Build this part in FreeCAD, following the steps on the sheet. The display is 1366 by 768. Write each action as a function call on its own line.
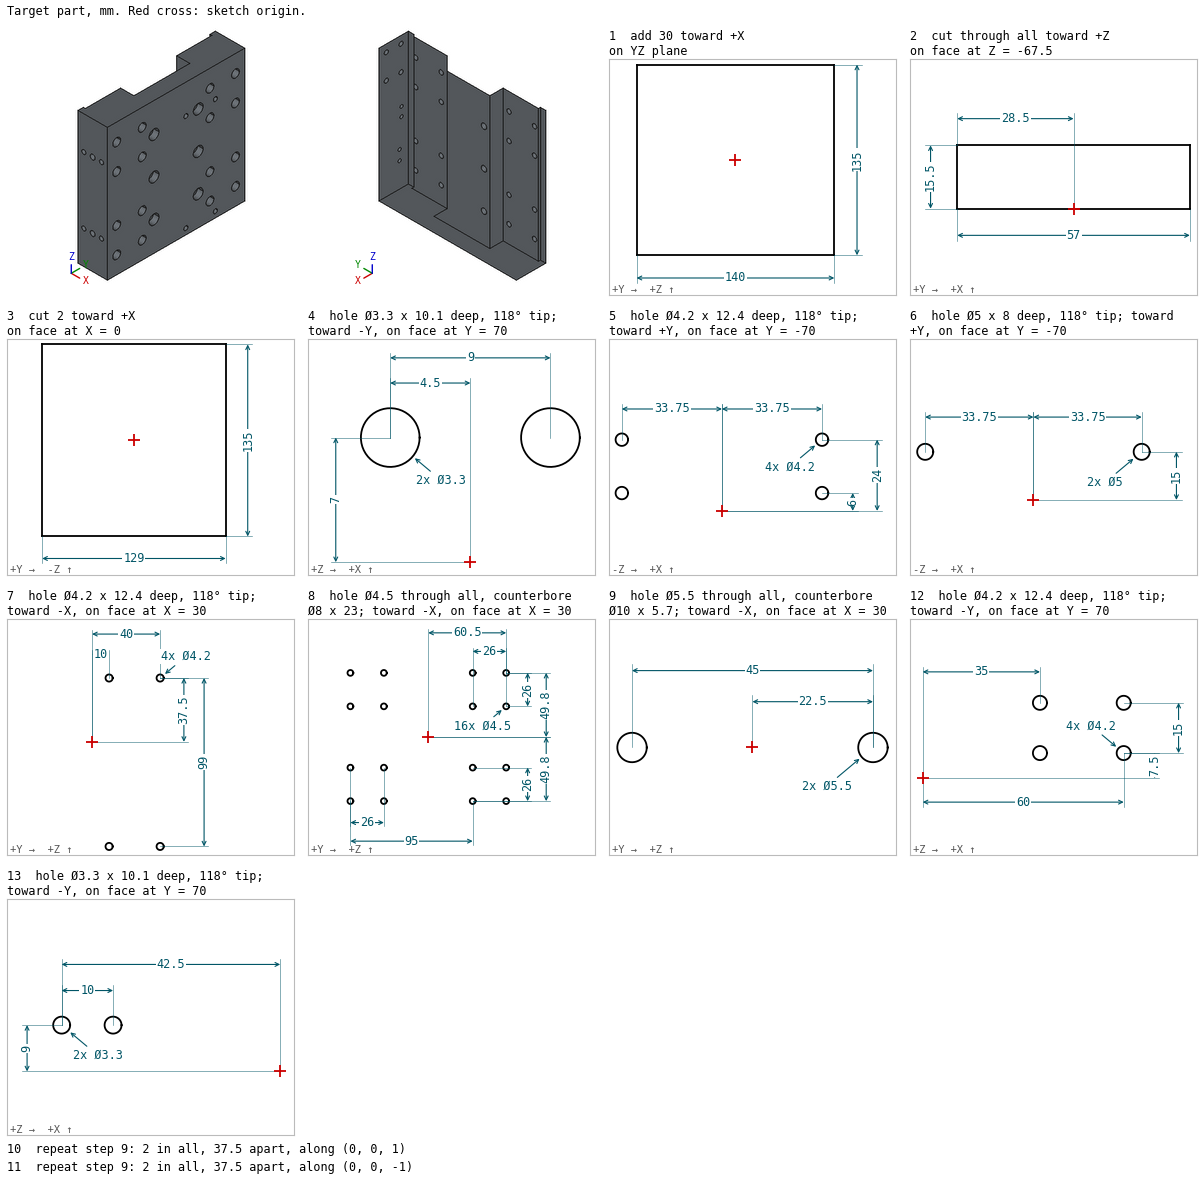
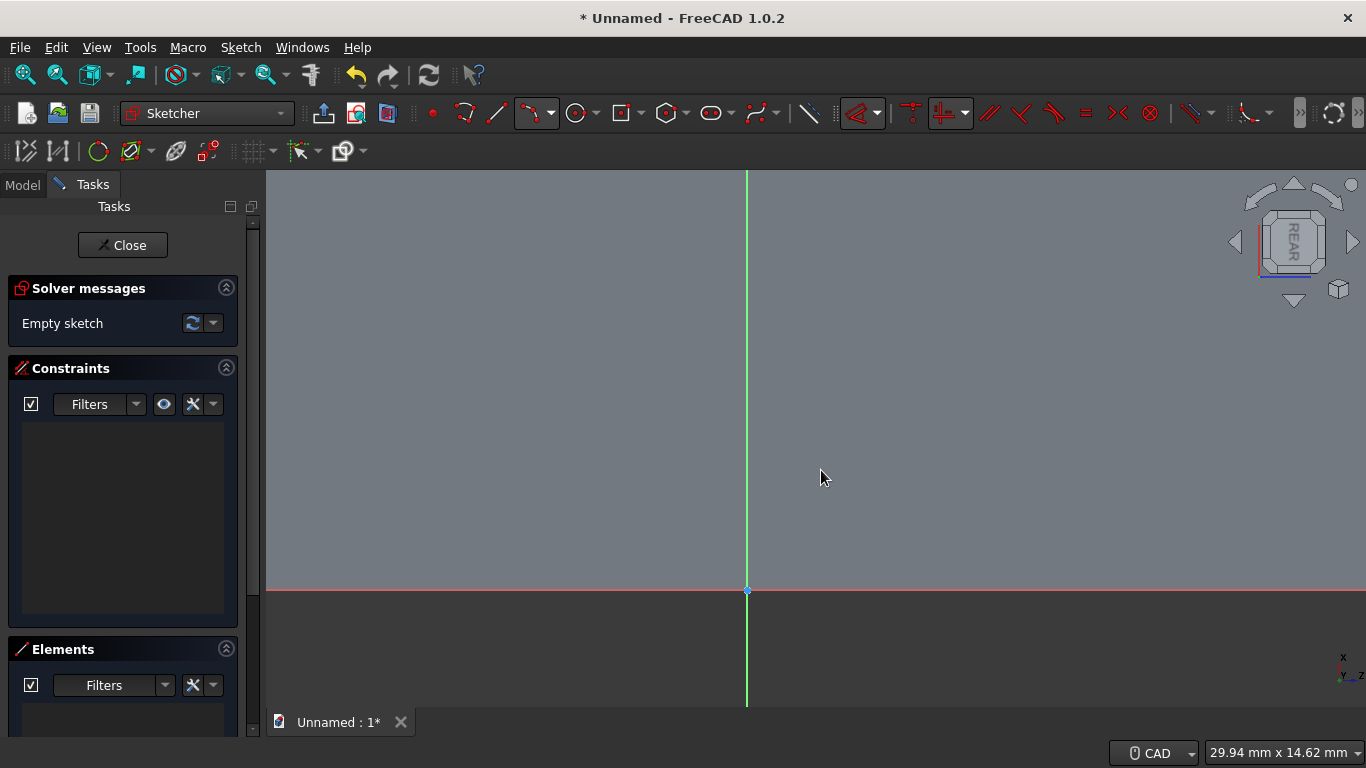
click(576, 114)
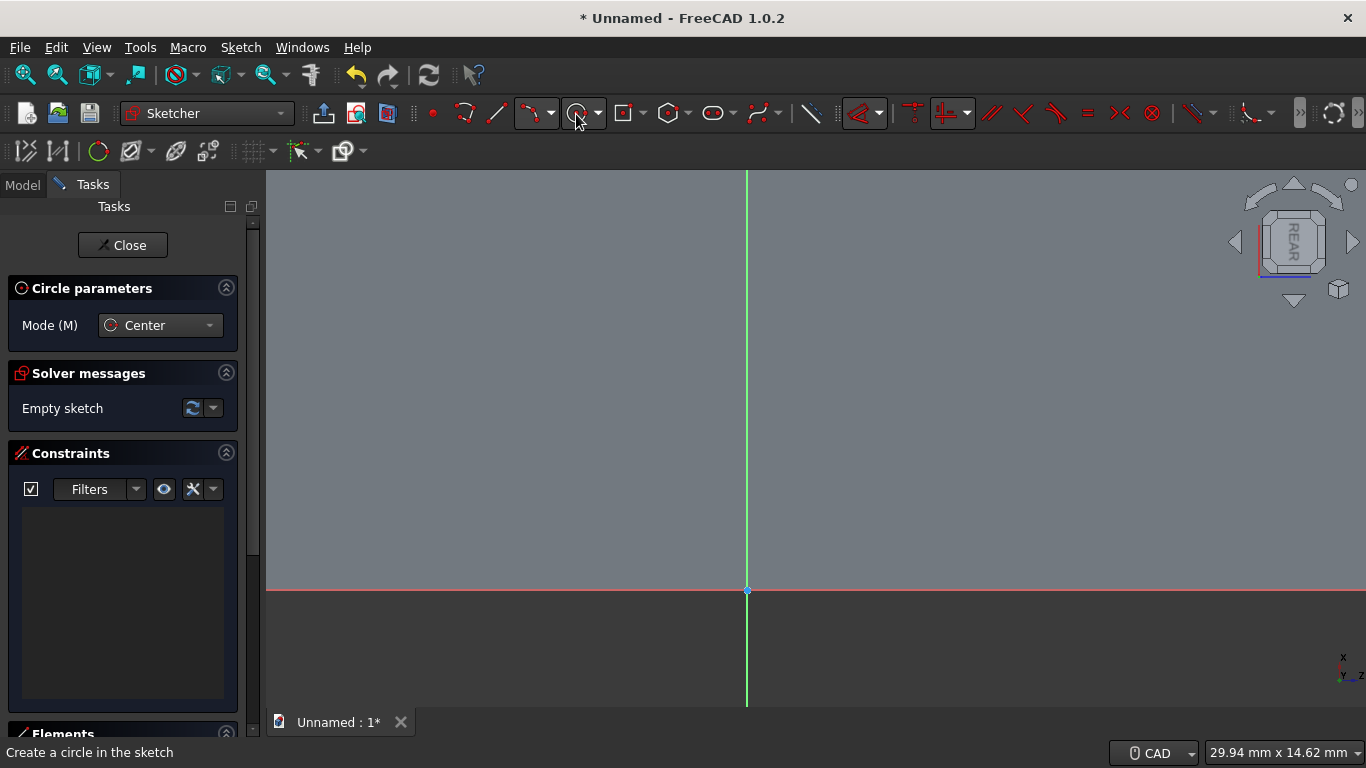
click(582, 333)
click(625, 290)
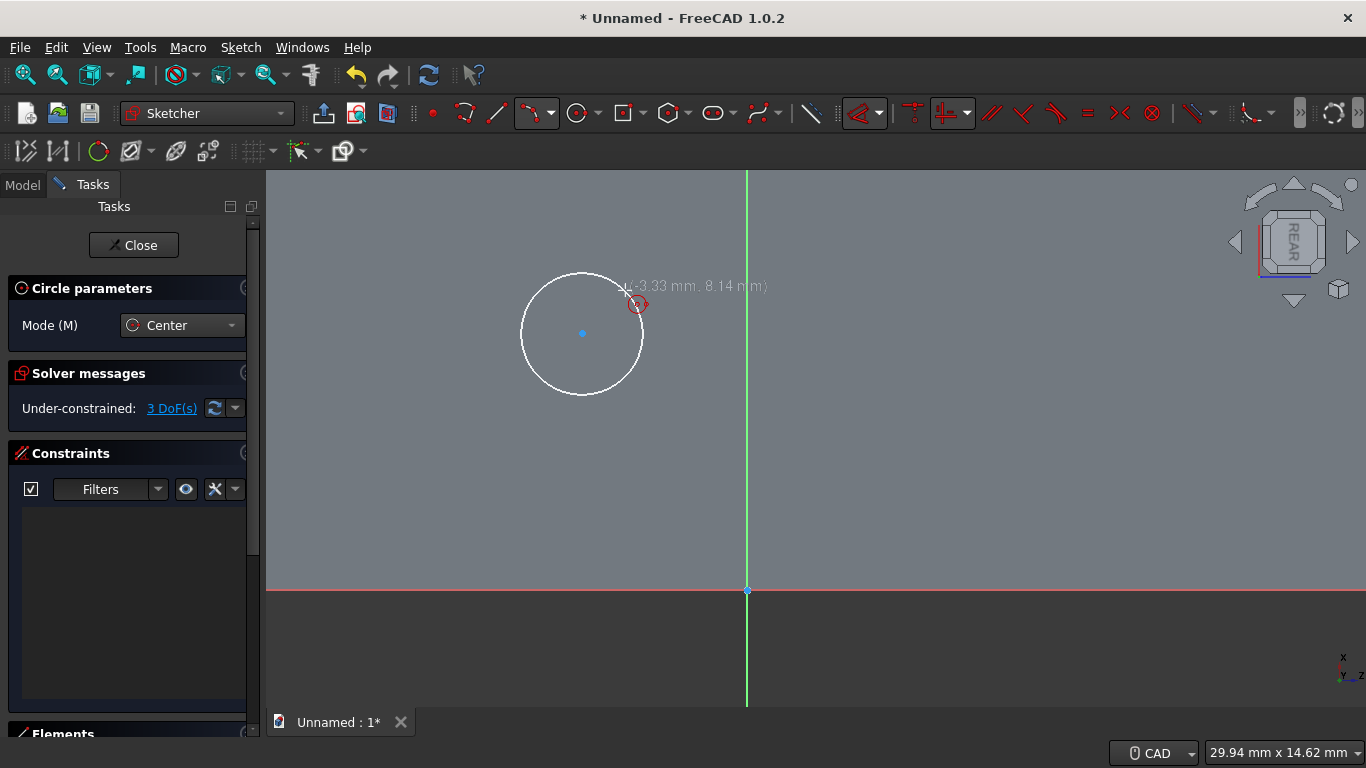
click(913, 333)
click(956, 290)
key(Escape)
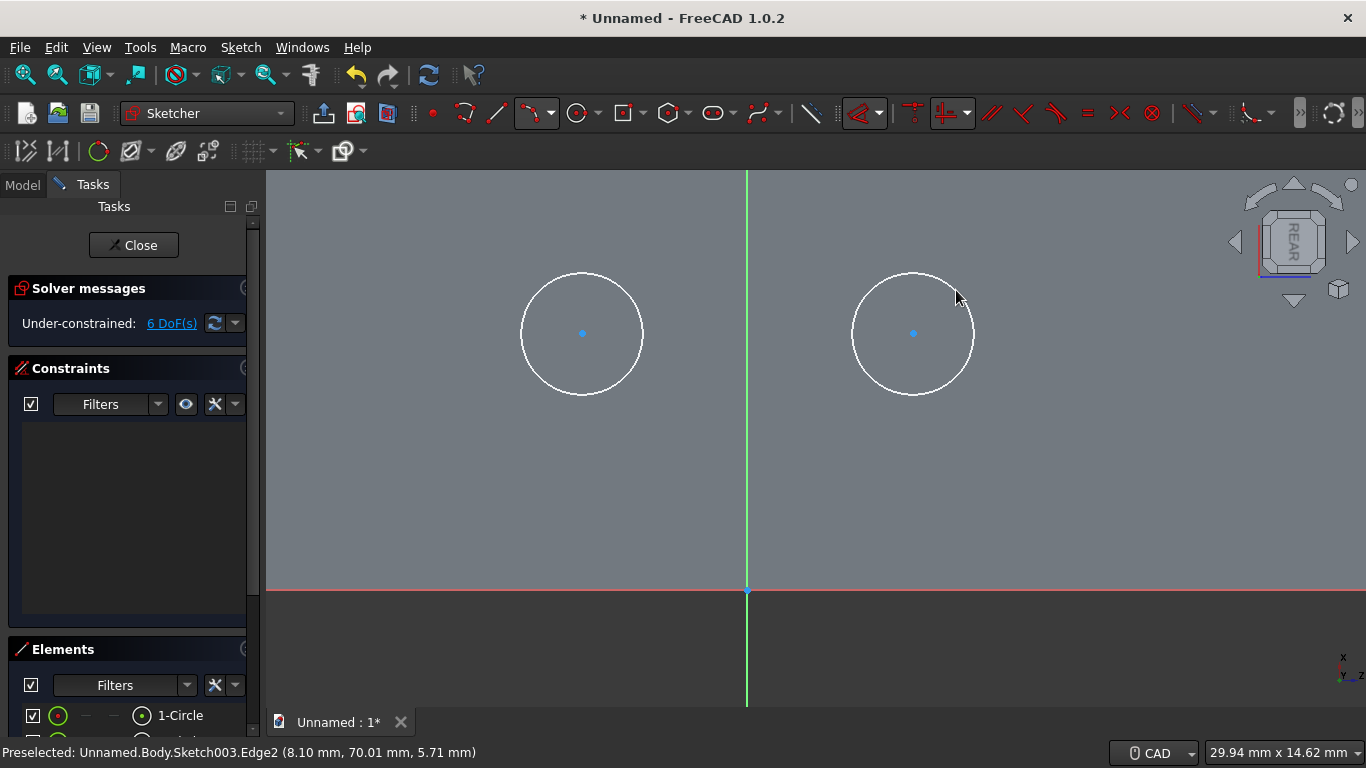
click(625, 291)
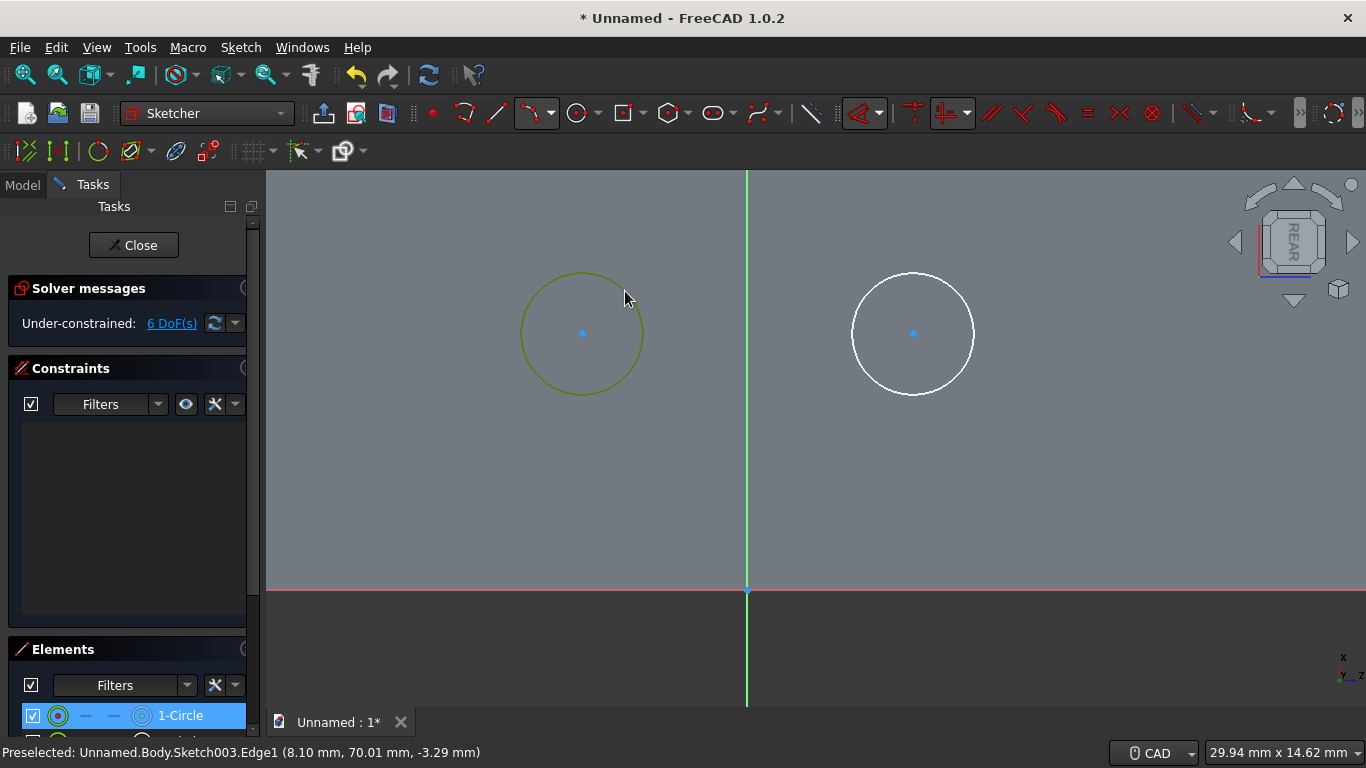
click(956, 291)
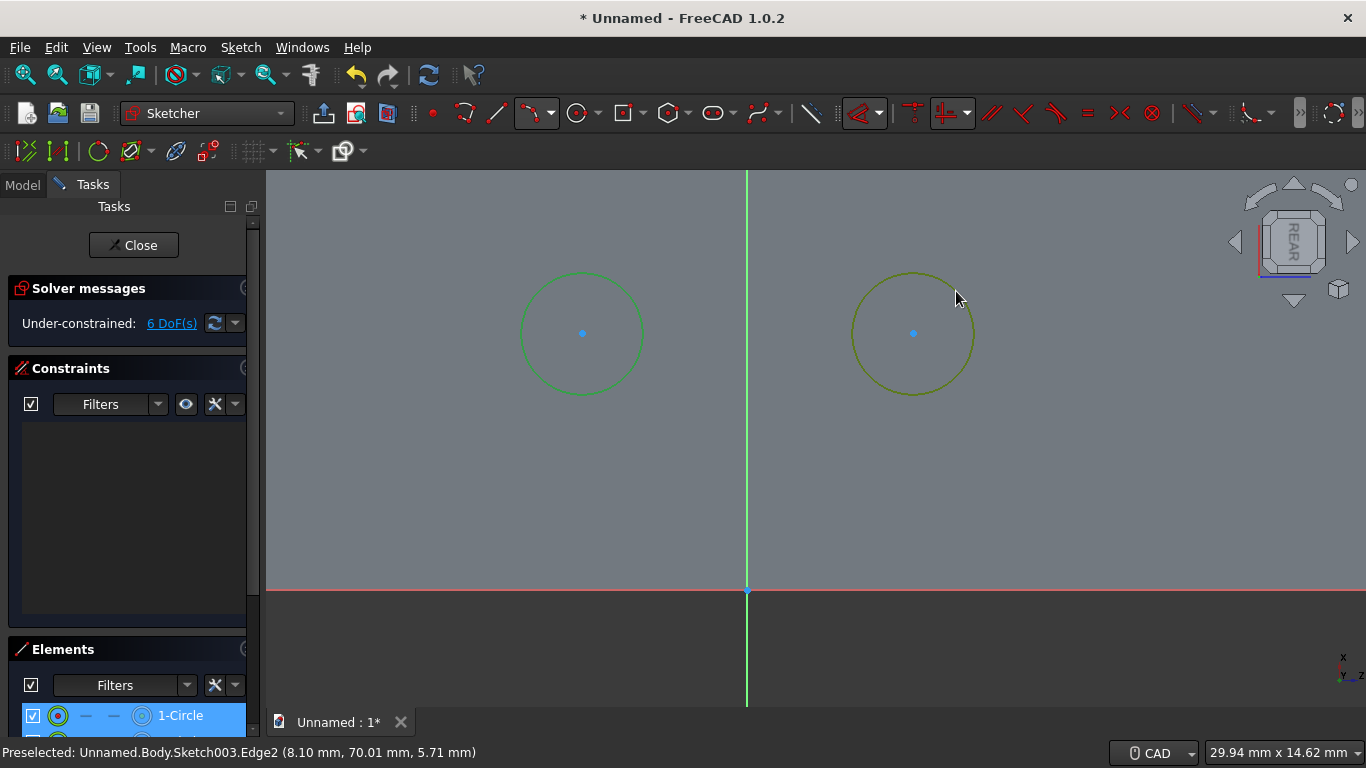
click(1088, 114)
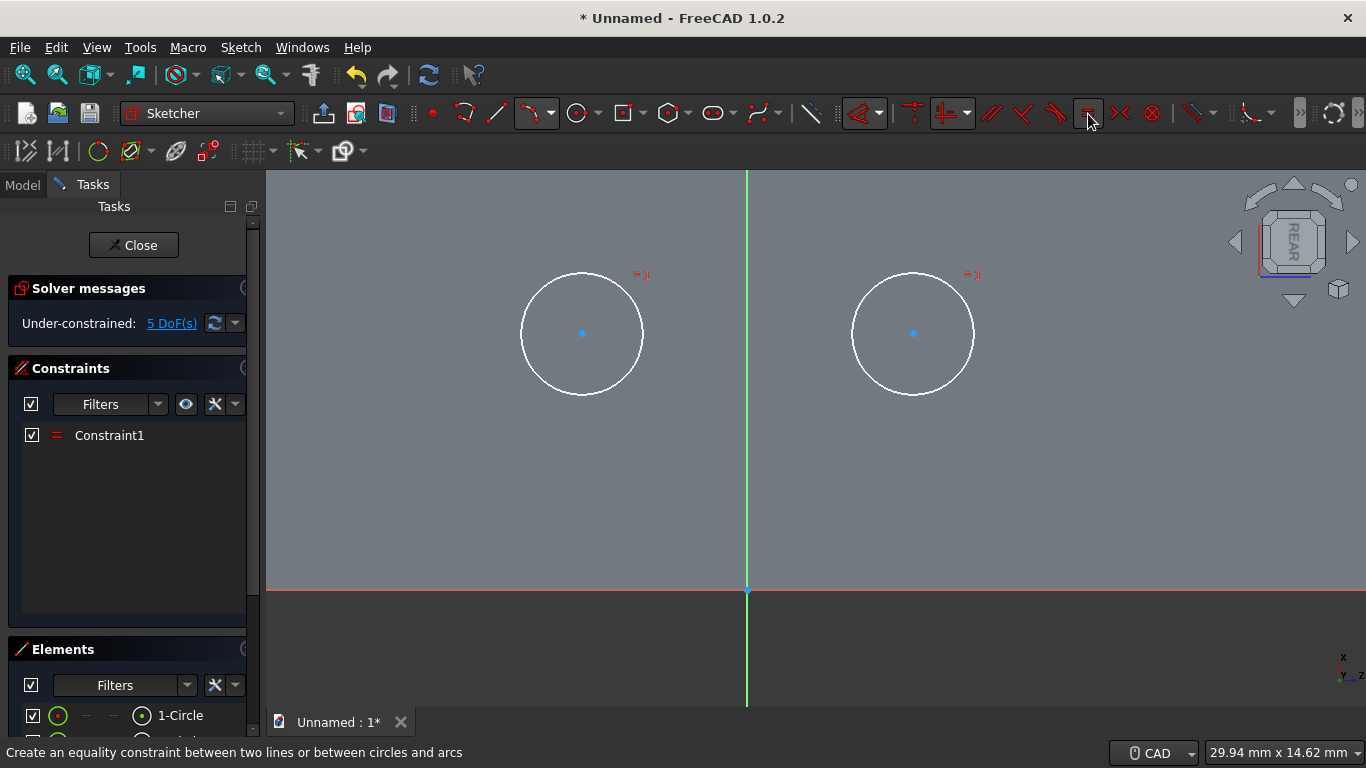
click(582, 334)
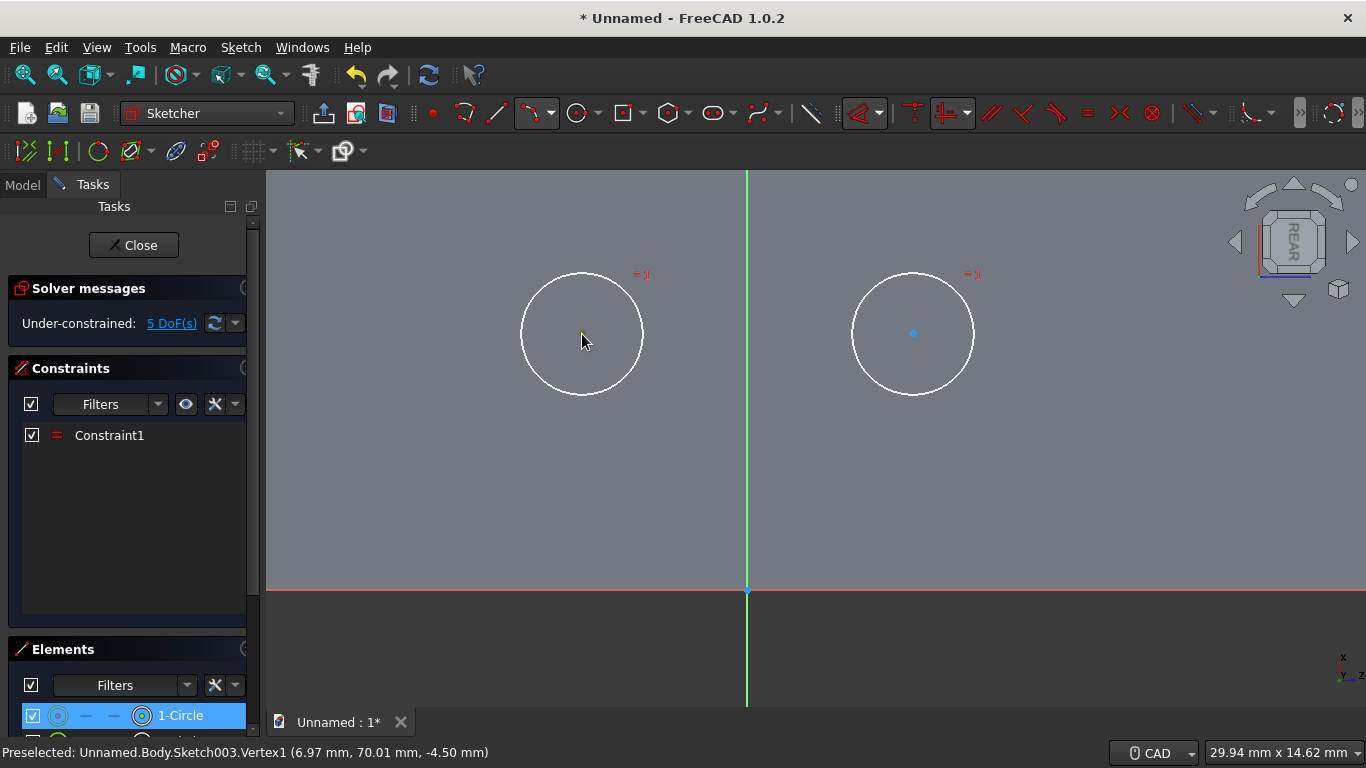
click(913, 334)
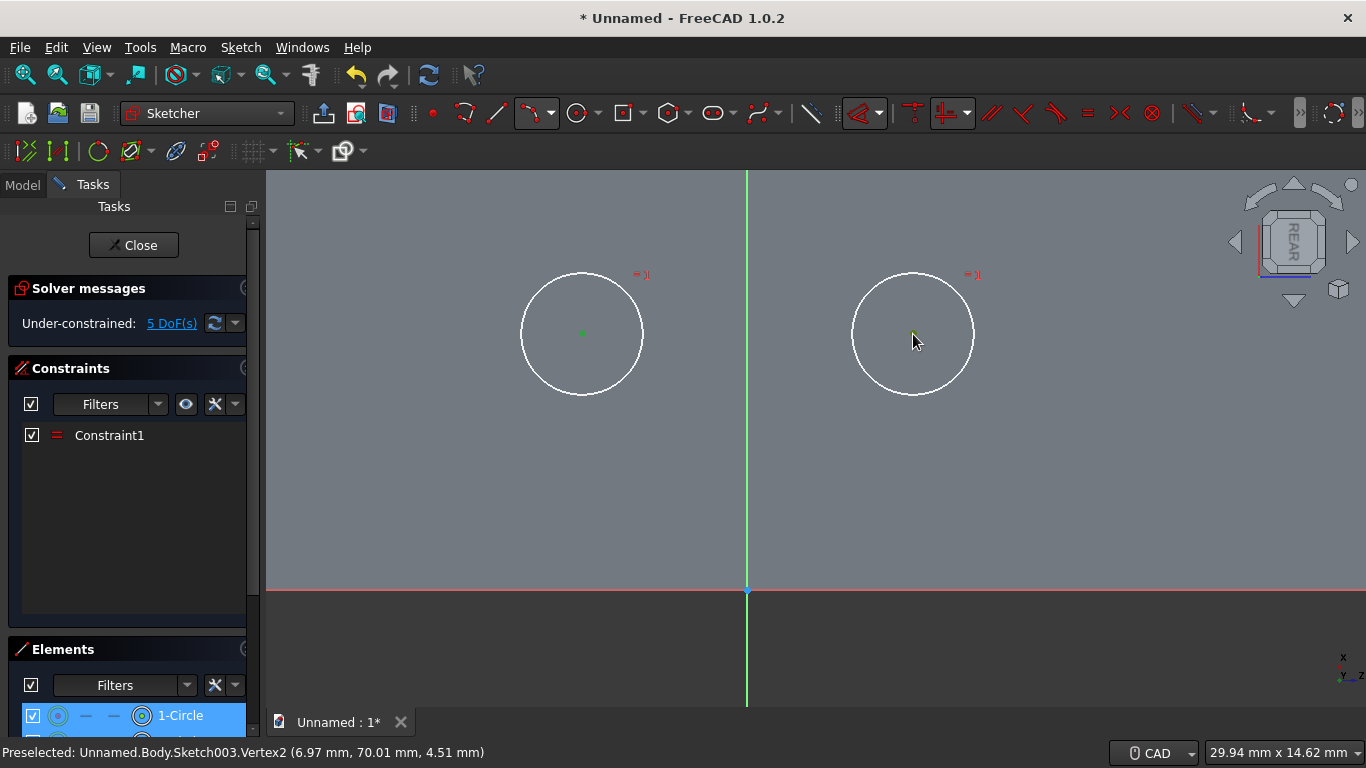
click(970, 114)